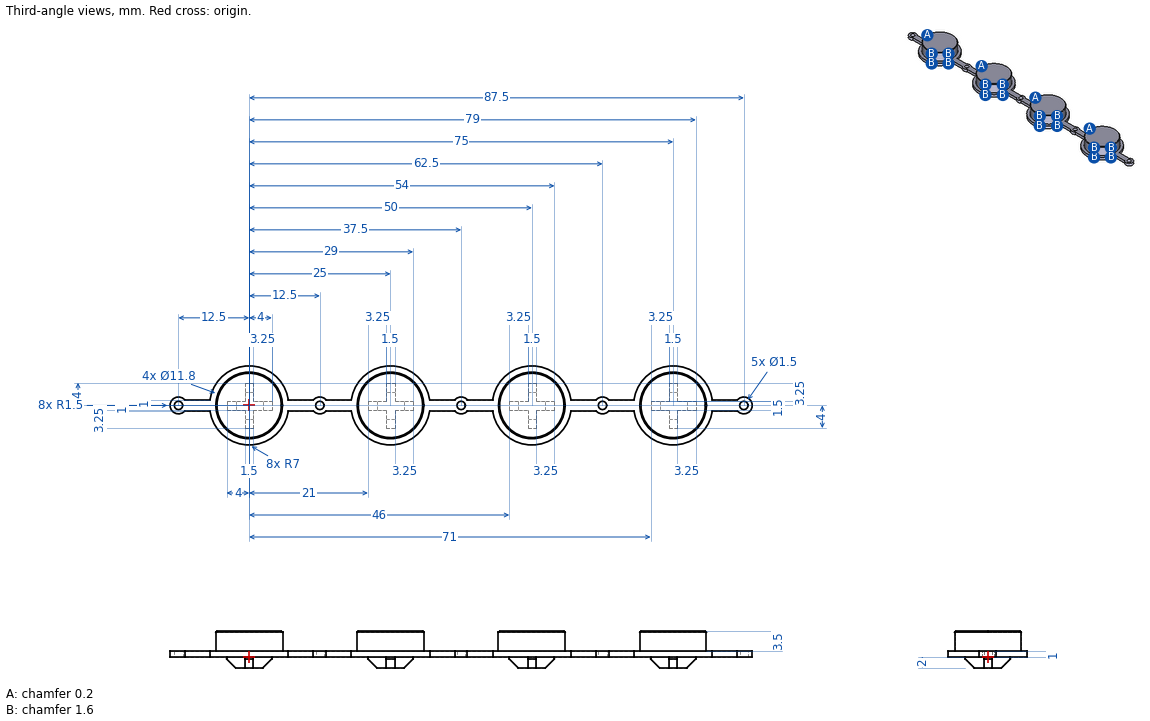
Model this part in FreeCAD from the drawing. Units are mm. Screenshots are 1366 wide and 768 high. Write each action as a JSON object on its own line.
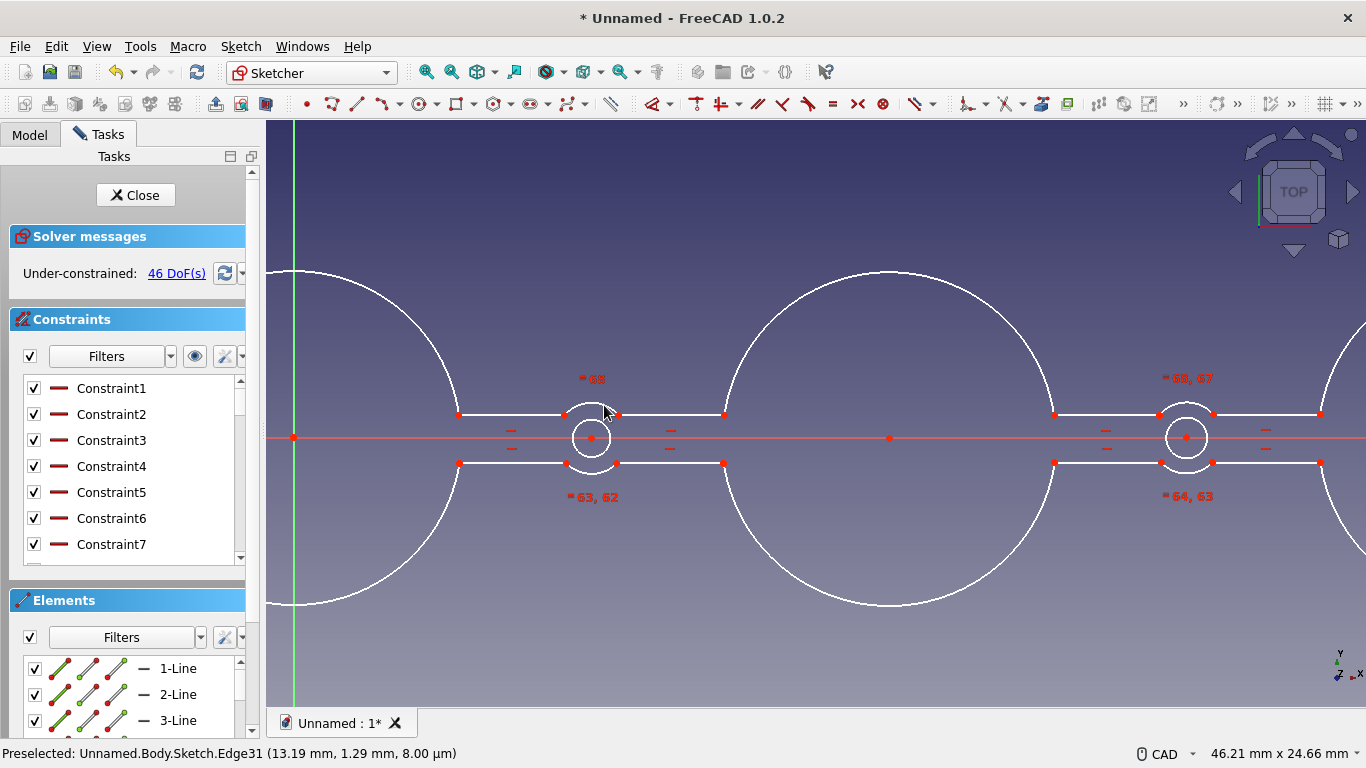
{"action": "scroll", "coordinate": [604, 406], "scroll_direction": "down", "scroll_amount": 7}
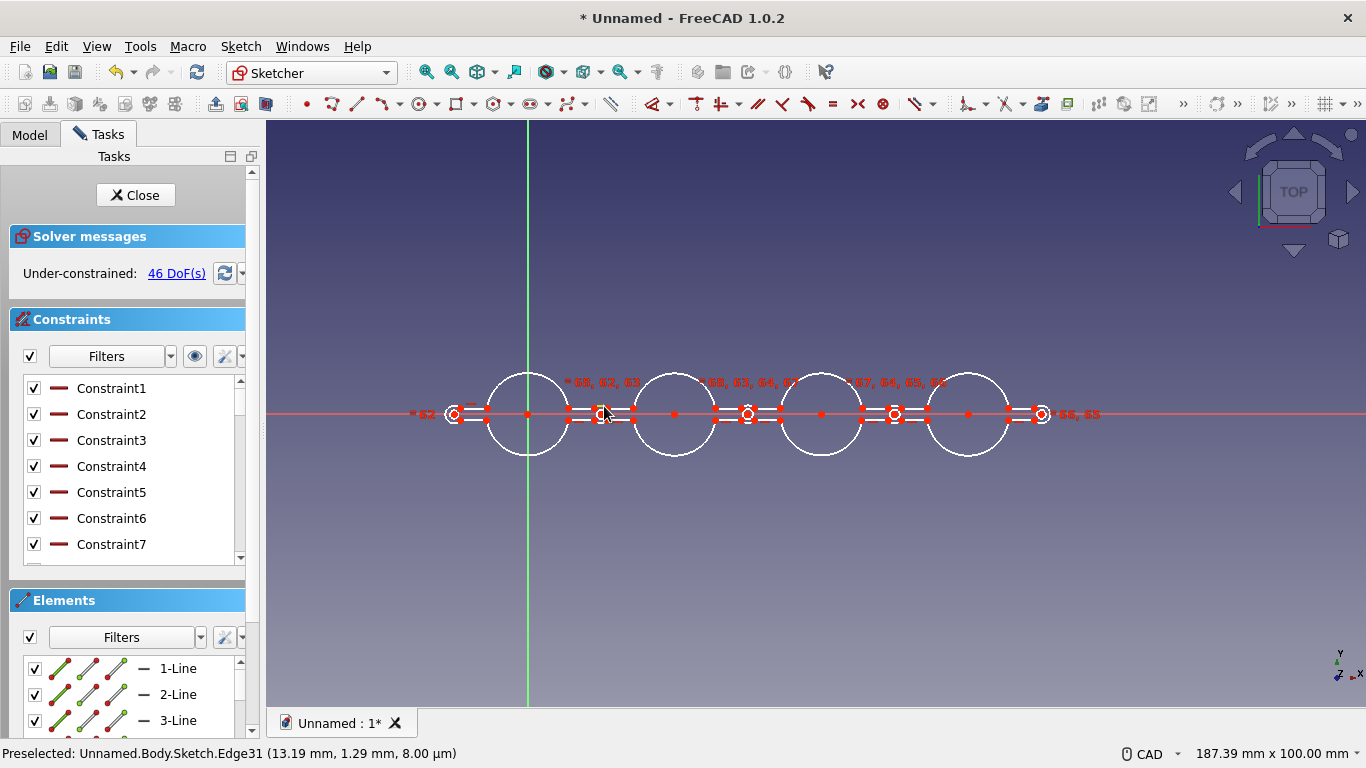
{"action": "left_click", "coordinate": [550, 449]}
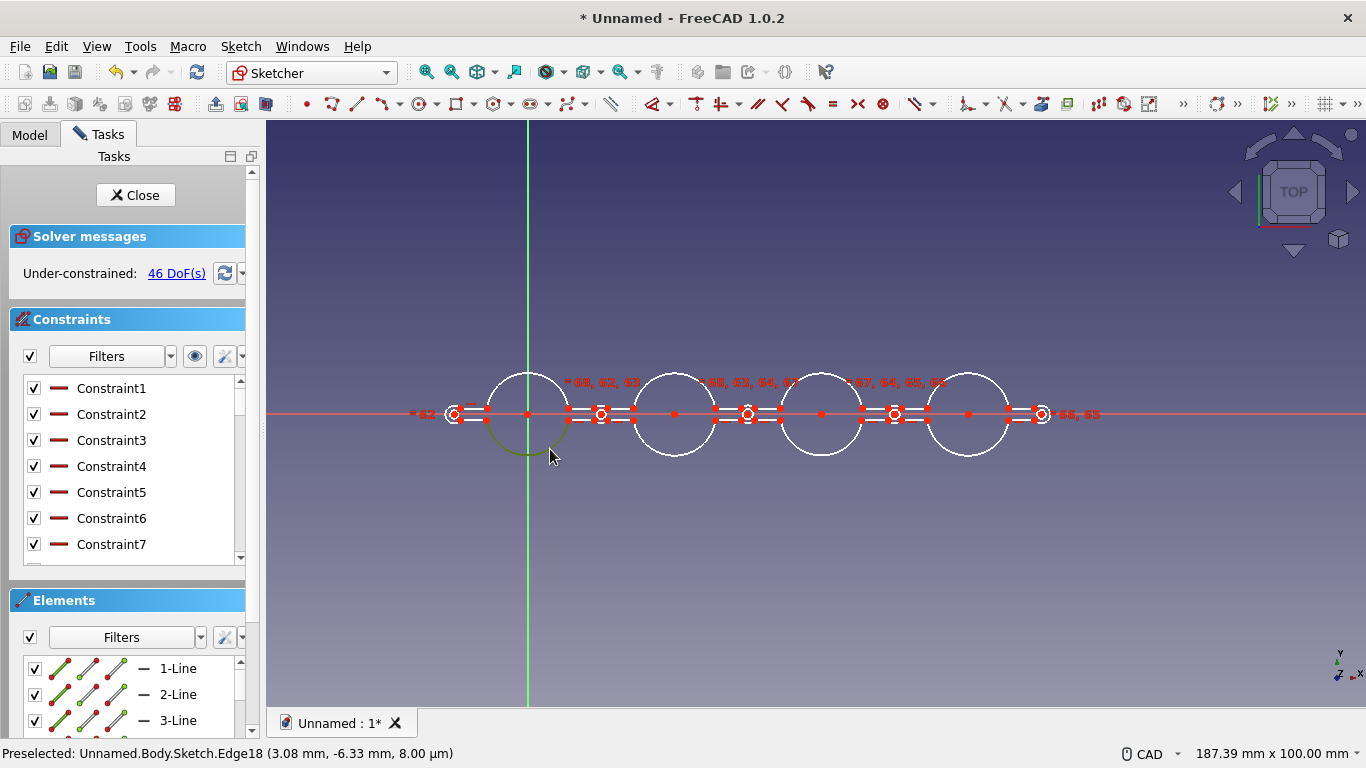
{"action": "left_click", "coordinate": [652, 449]}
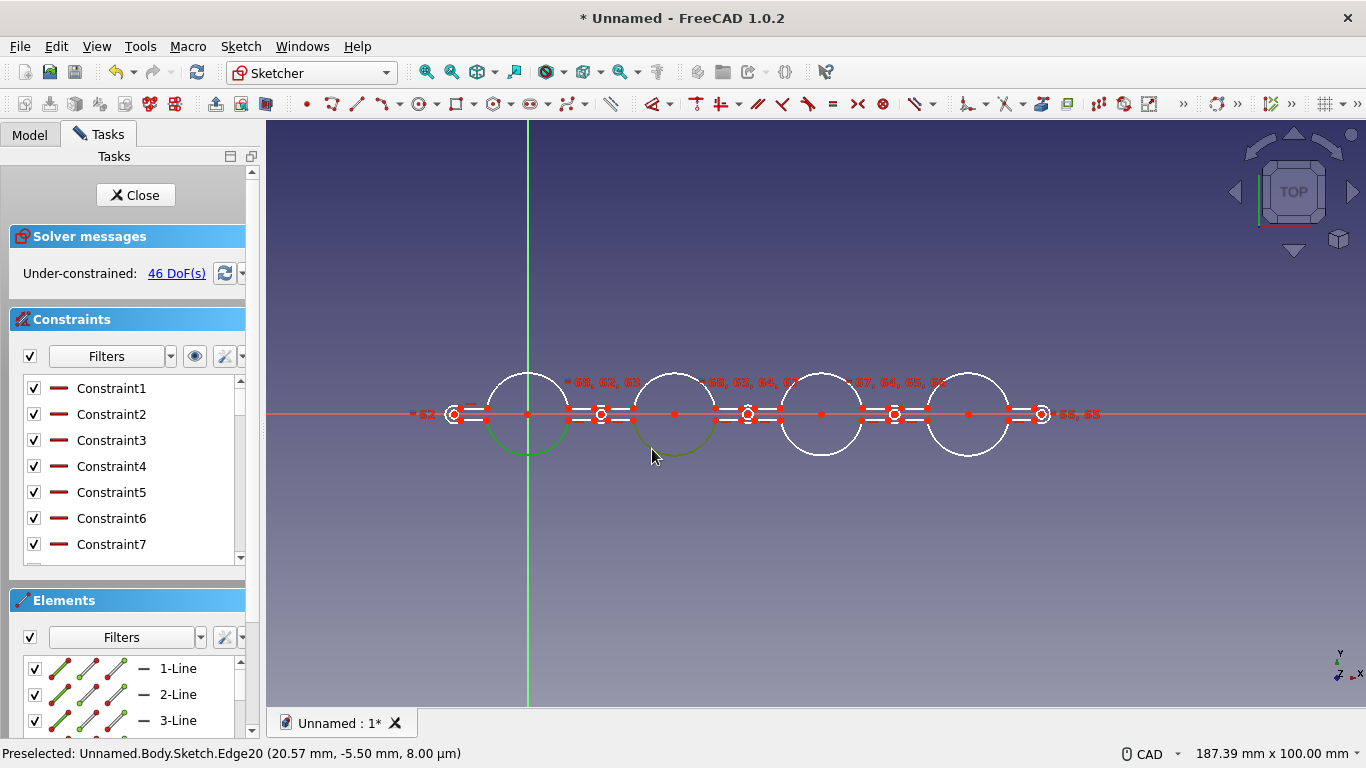
{"action": "left_click", "coordinate": [799, 449]}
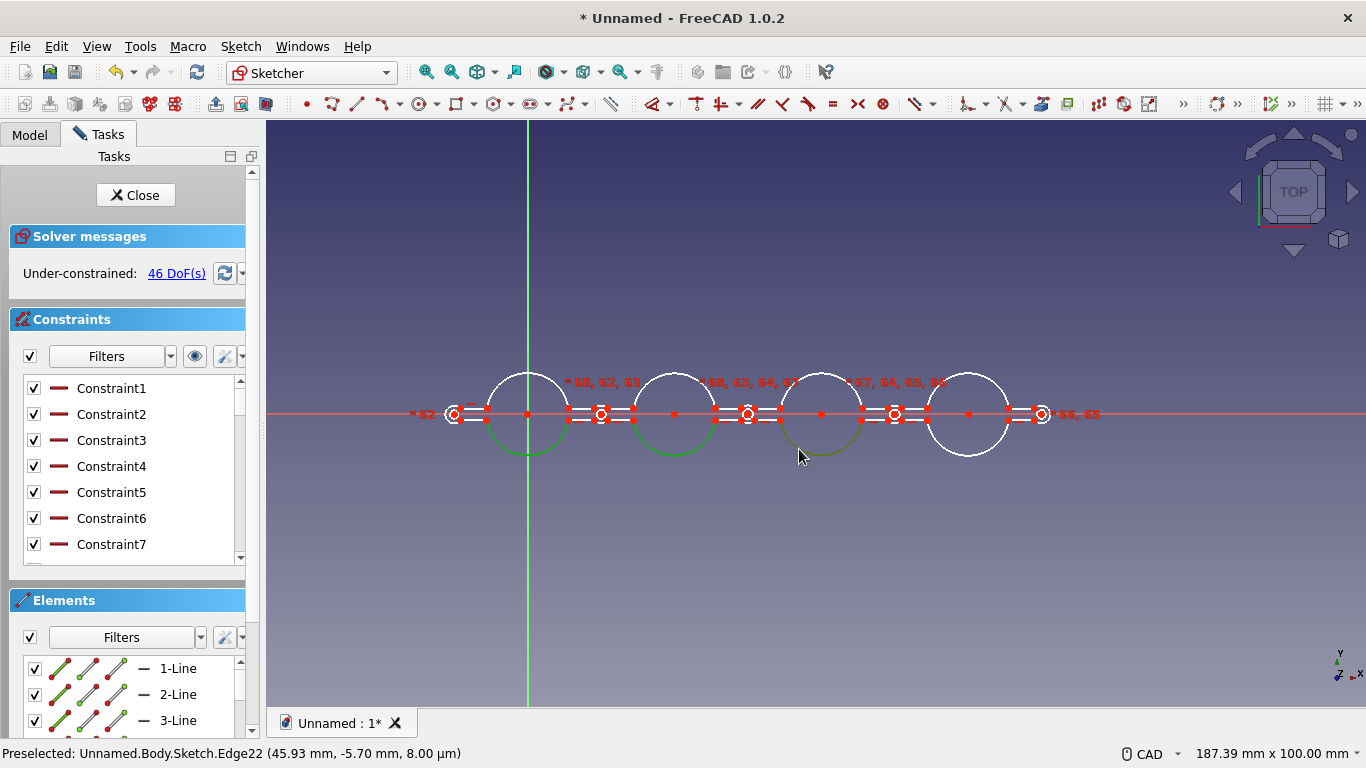
{"action": "left_click", "coordinate": [946, 449]}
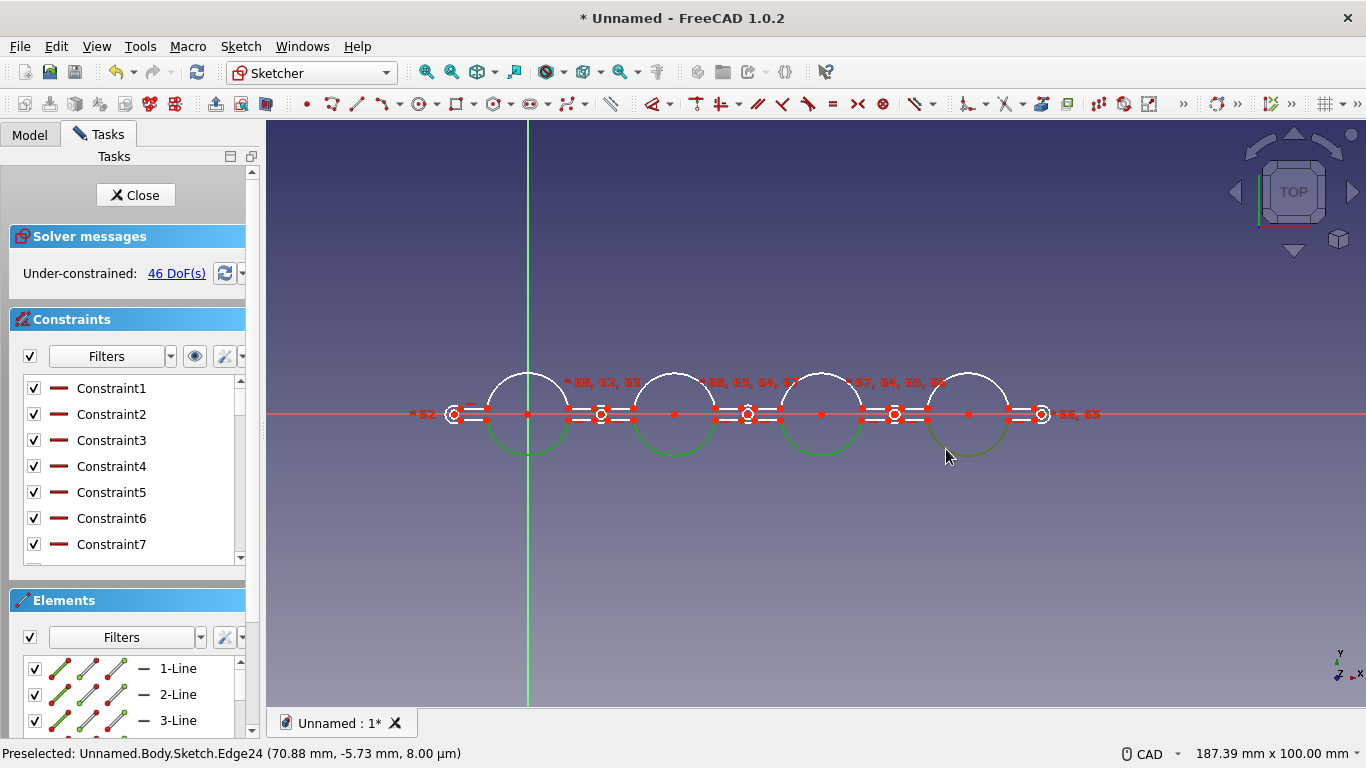
{"action": "left_click", "coordinate": [990, 380]}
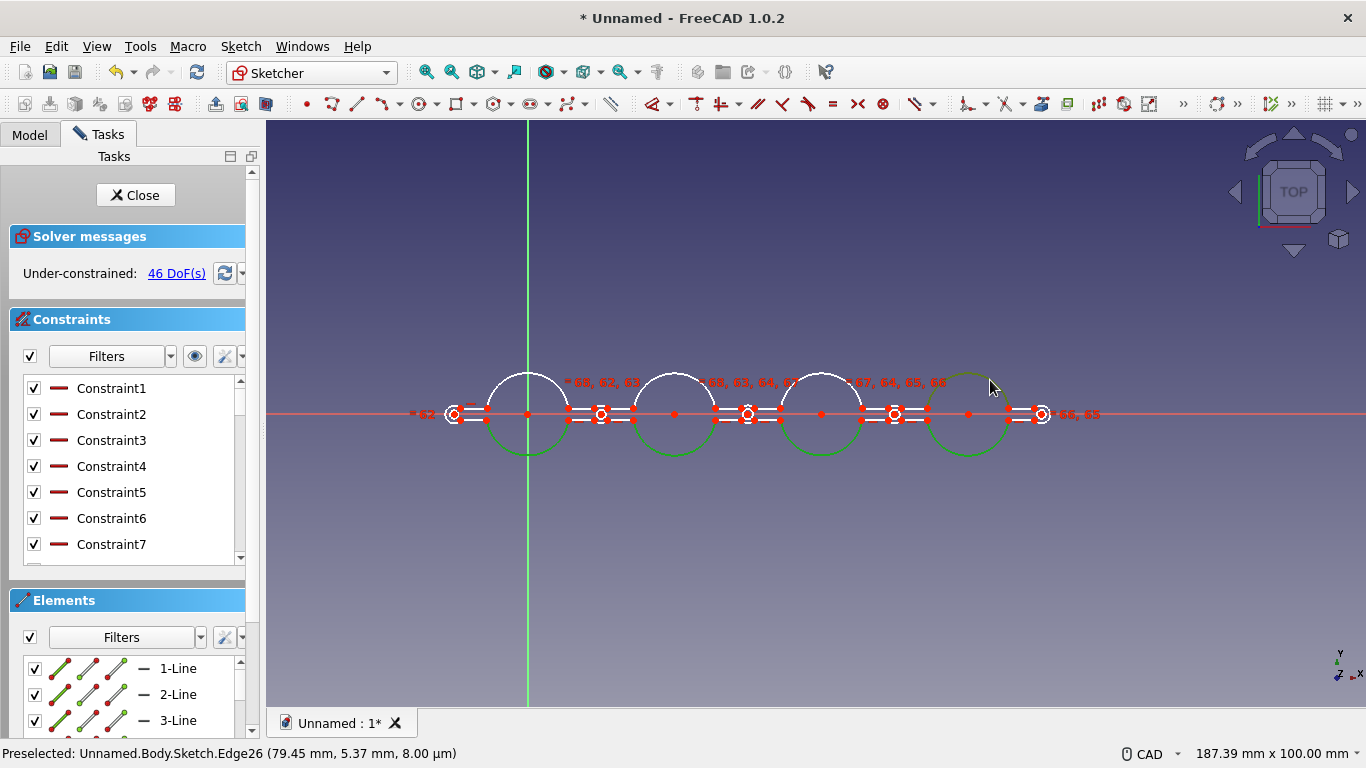
{"action": "left_click", "coordinate": [821, 373]}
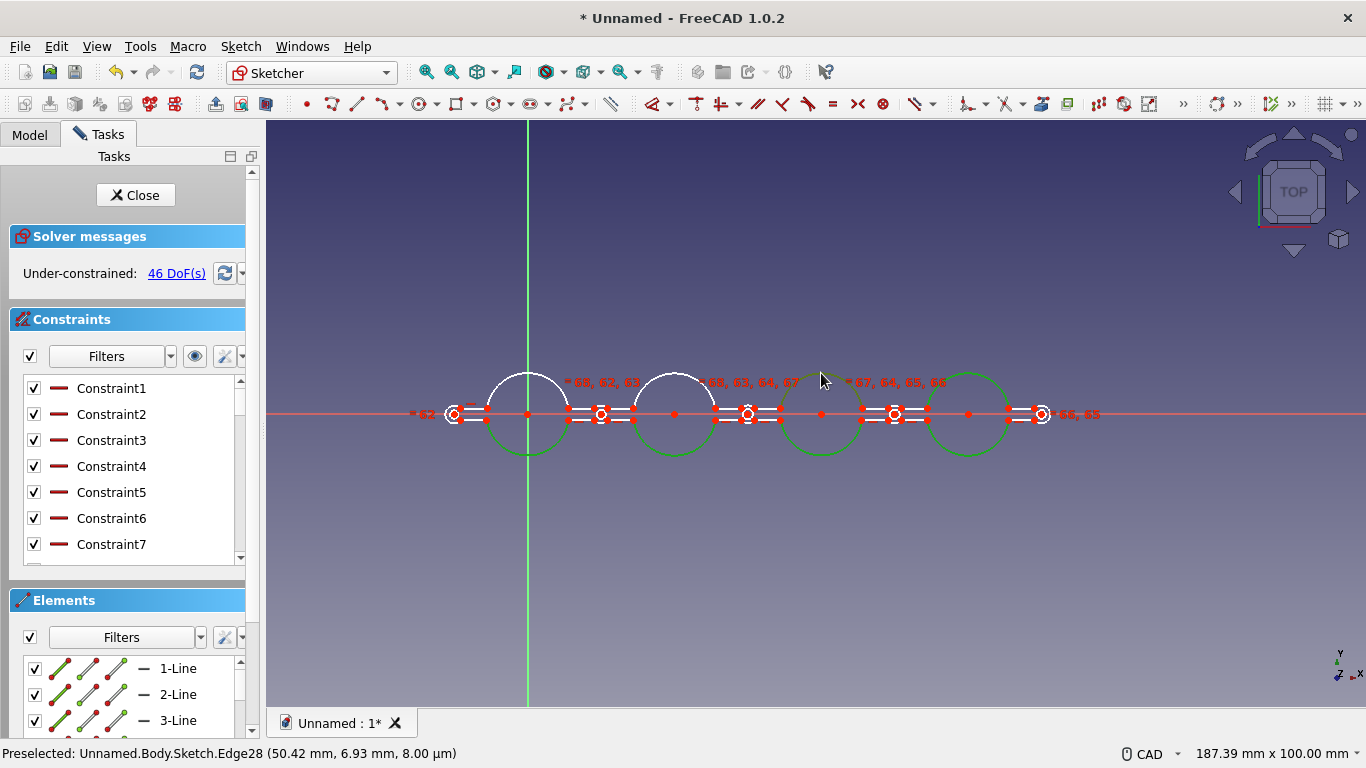
{"action": "left_click", "coordinate": [652, 380]}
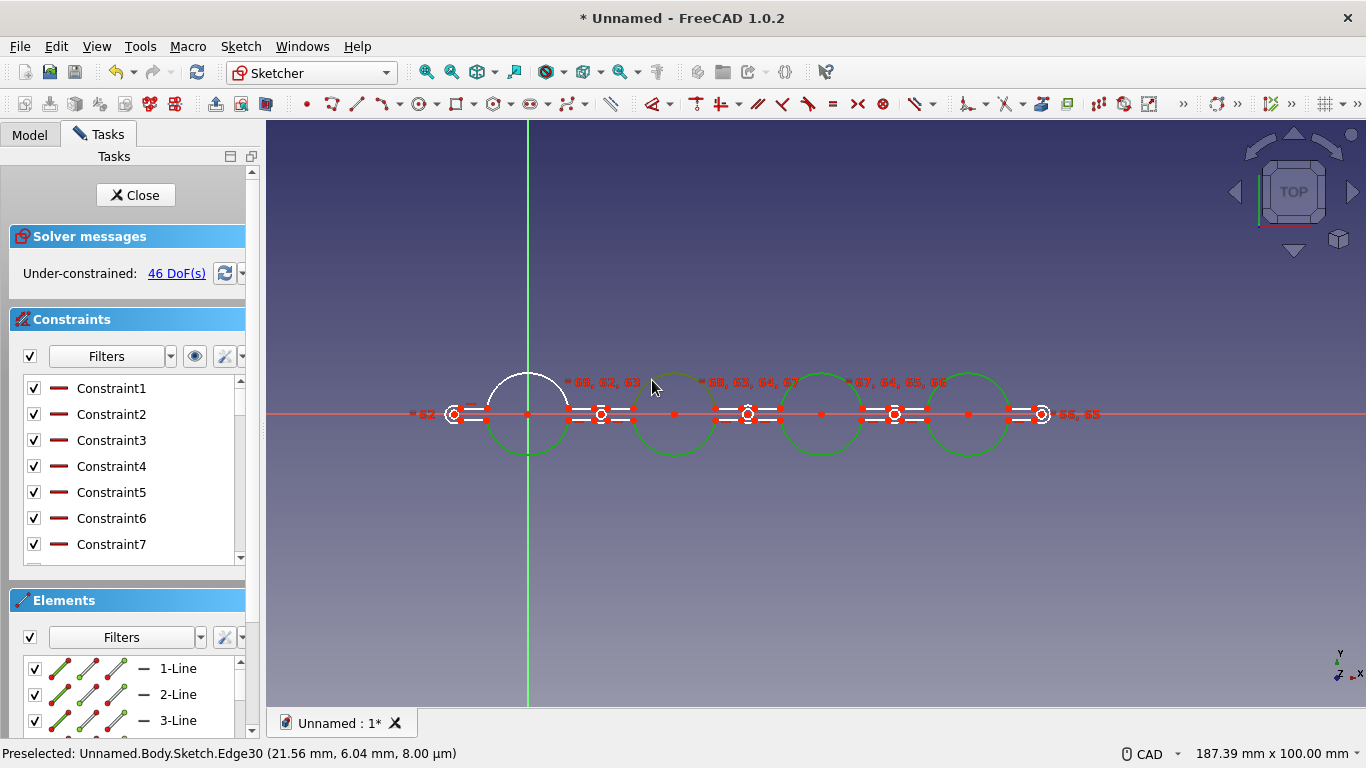
{"action": "left_click", "coordinate": [550, 380]}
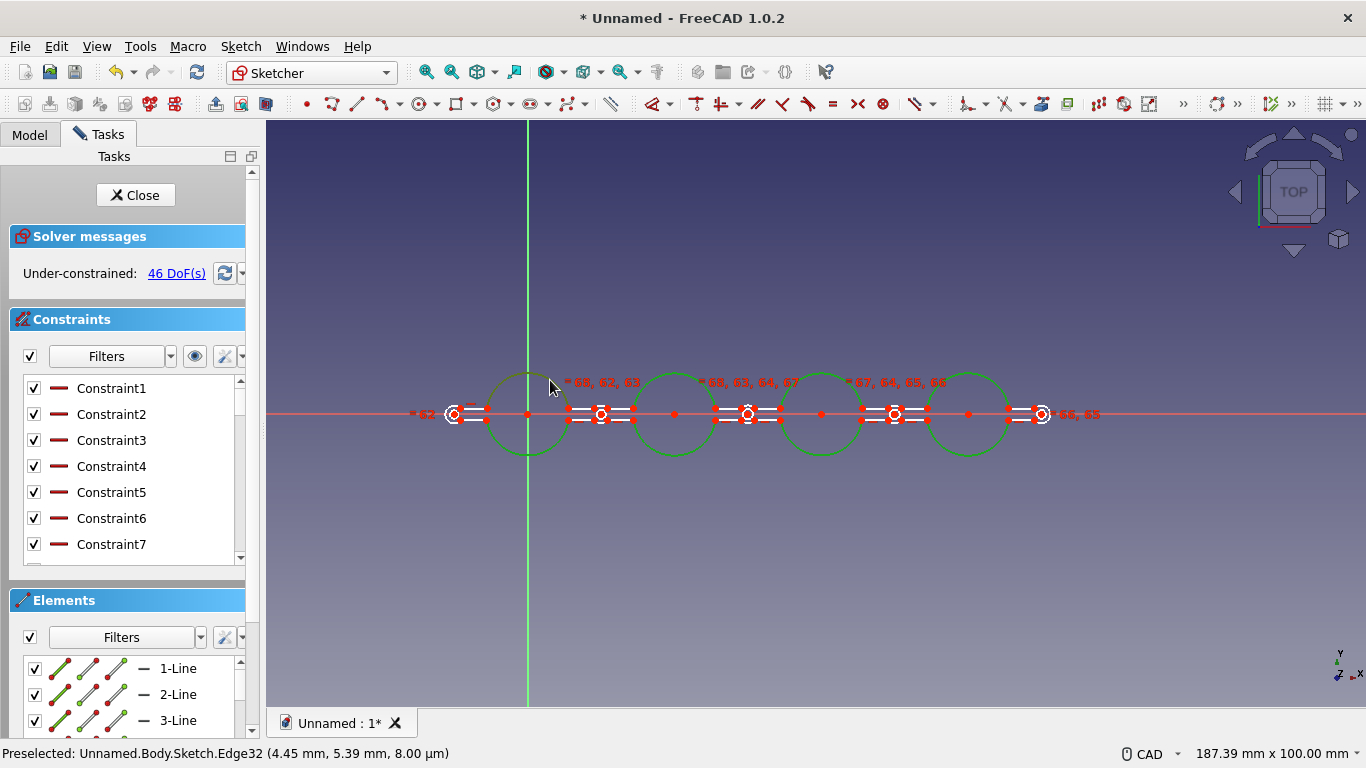
{"action": "left_click", "coordinate": [833, 104]}